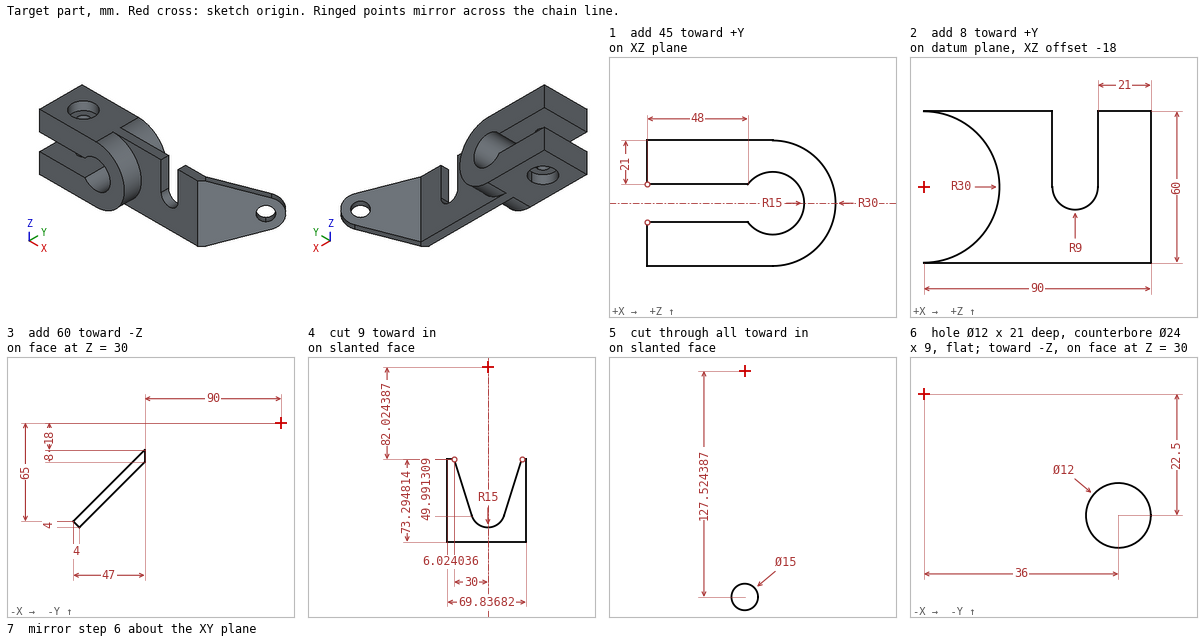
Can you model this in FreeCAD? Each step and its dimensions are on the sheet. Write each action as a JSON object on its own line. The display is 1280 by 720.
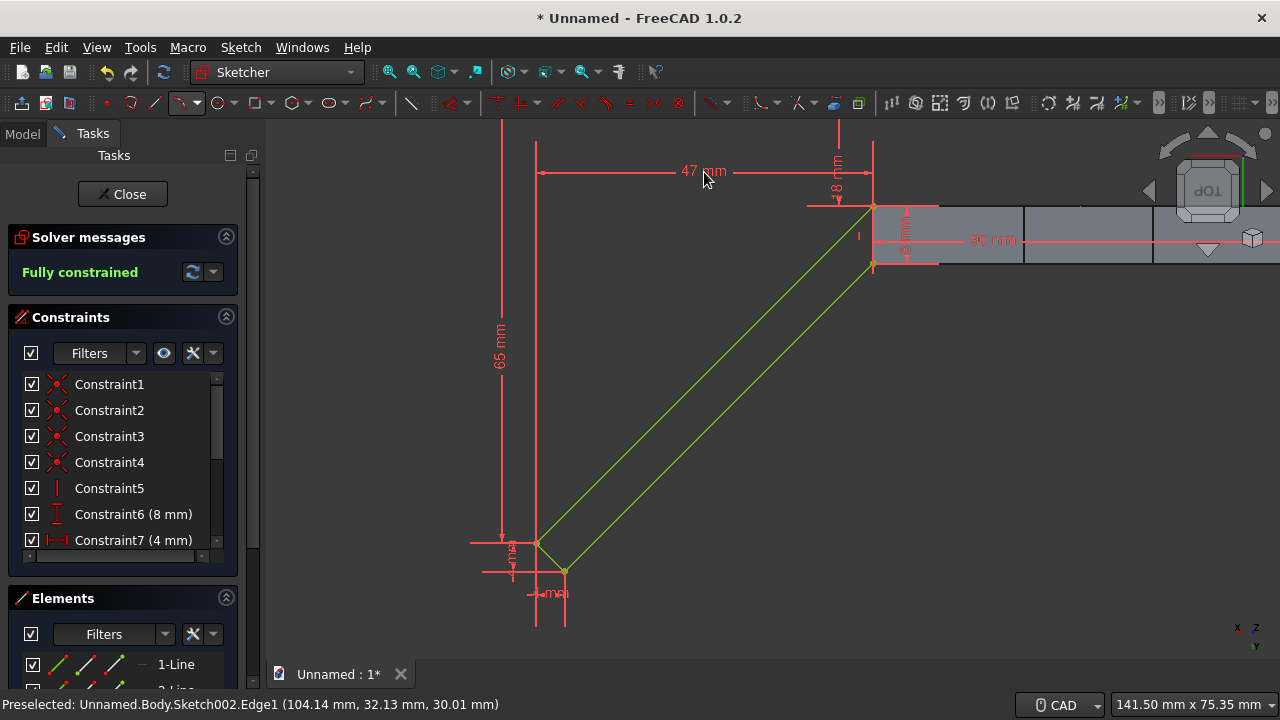
{"action": "left_click", "coordinate": [123, 194]}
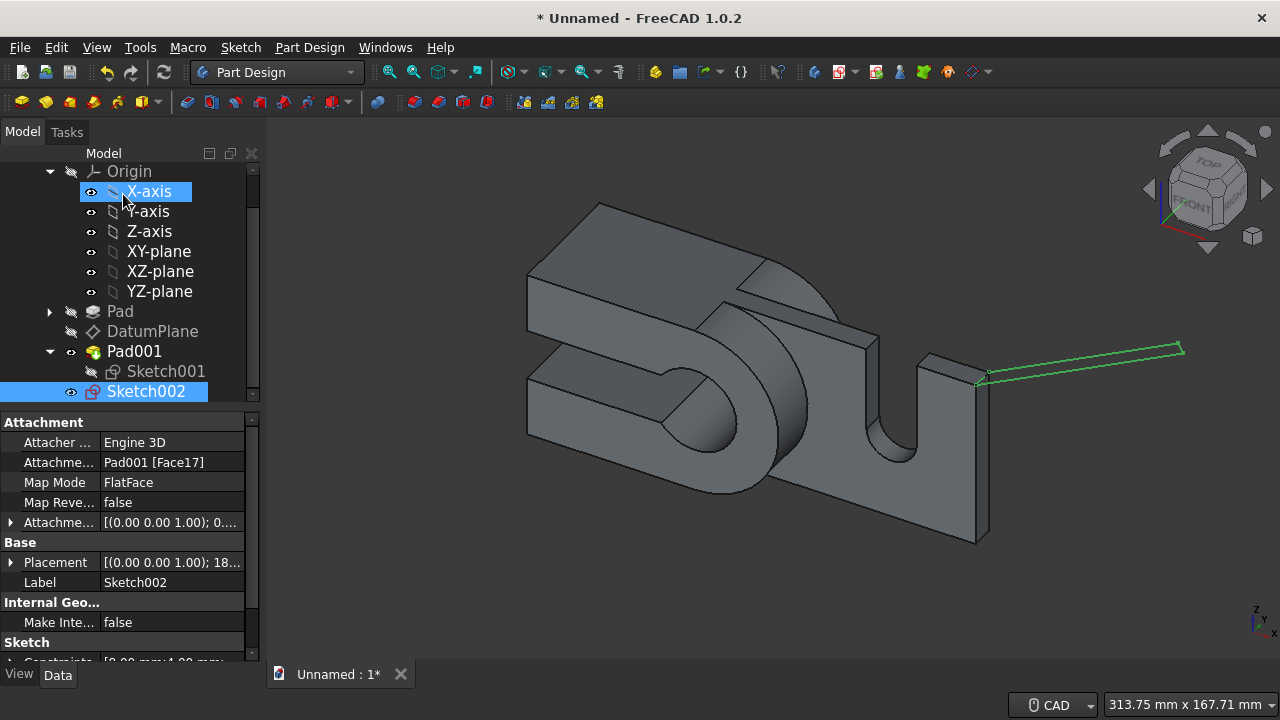
{"action": "left_click", "coordinate": [22, 102]}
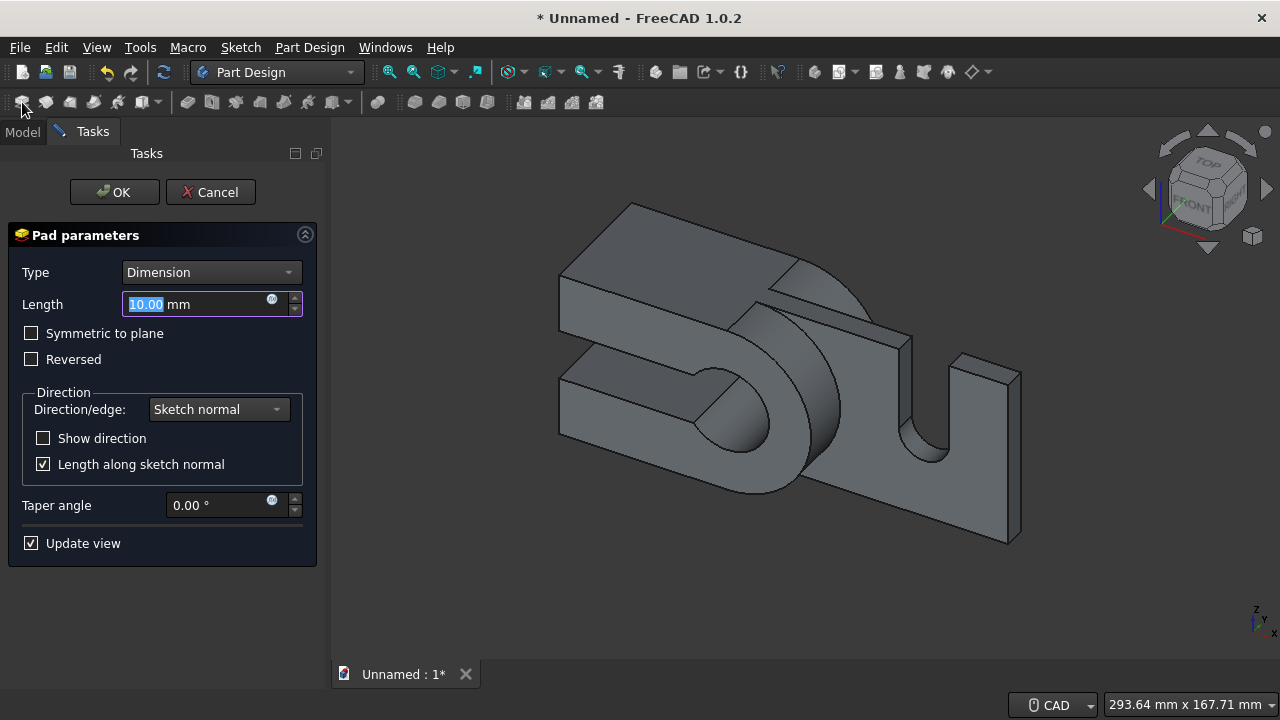
{"action": "type", "text": "60"}
{"action": "key", "text": "Tab"}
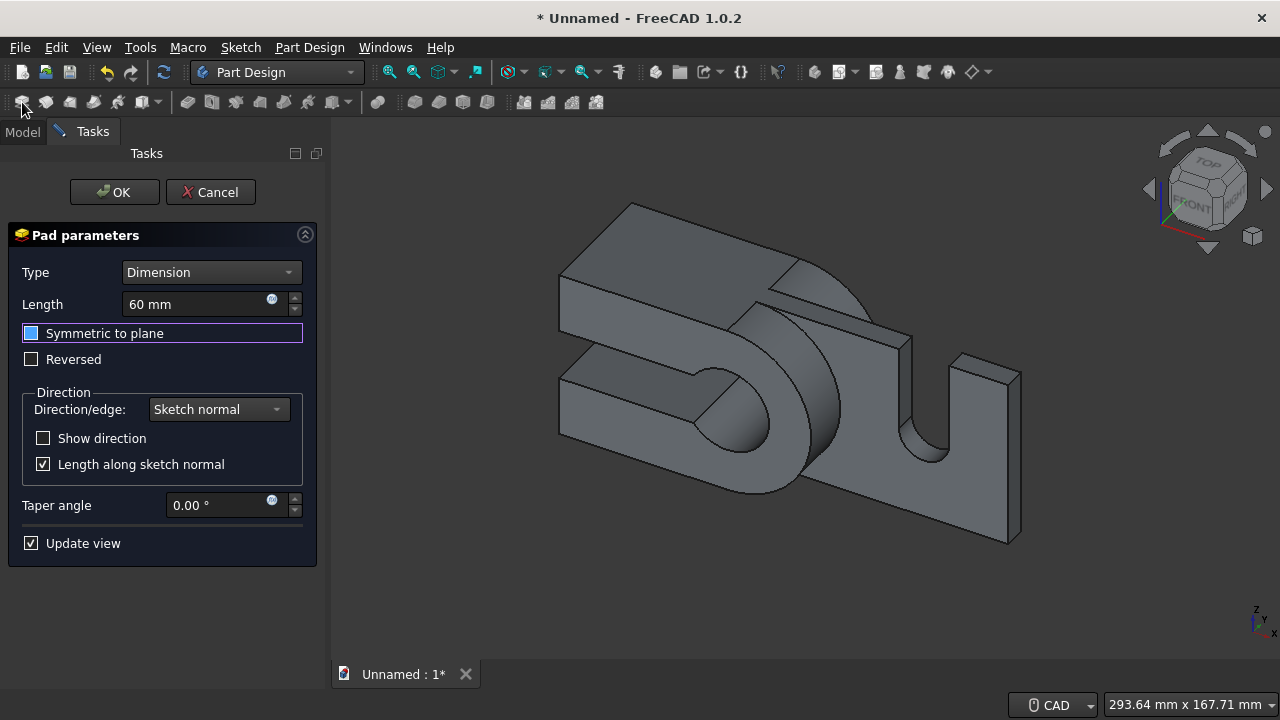
{"action": "left_click", "coordinate": [30, 359]}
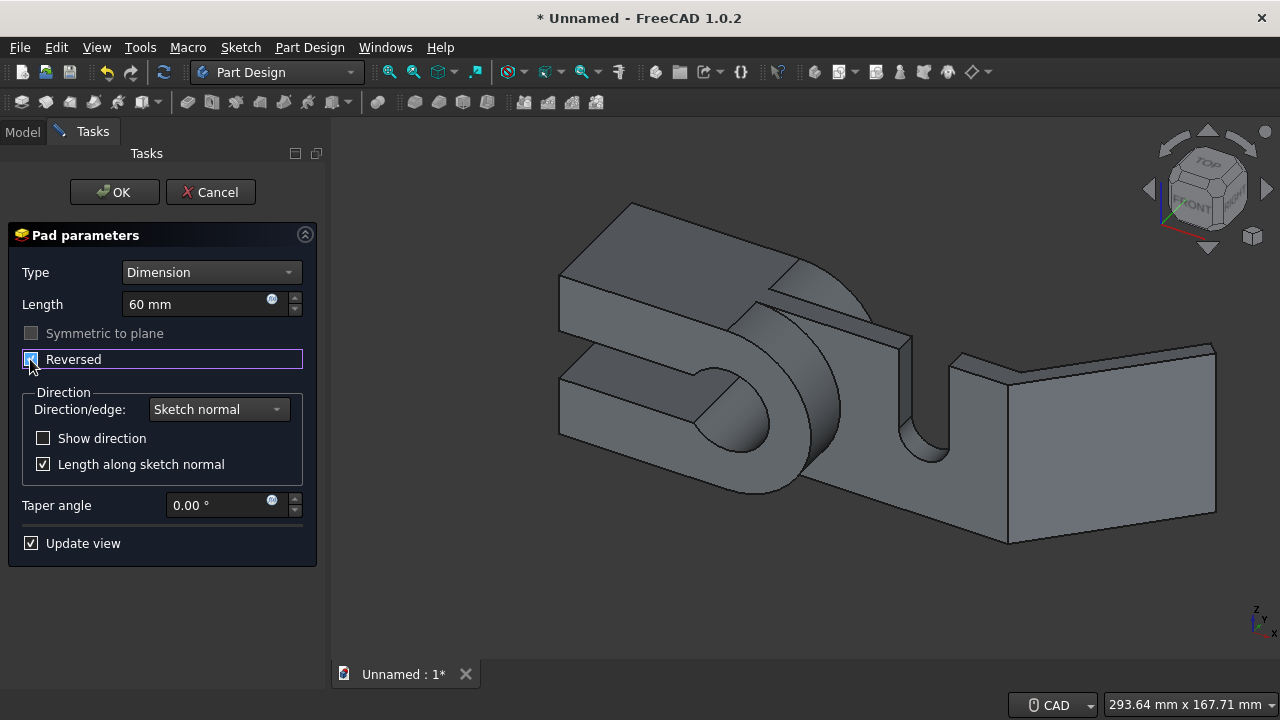
{"action": "left_click", "coordinate": [115, 192]}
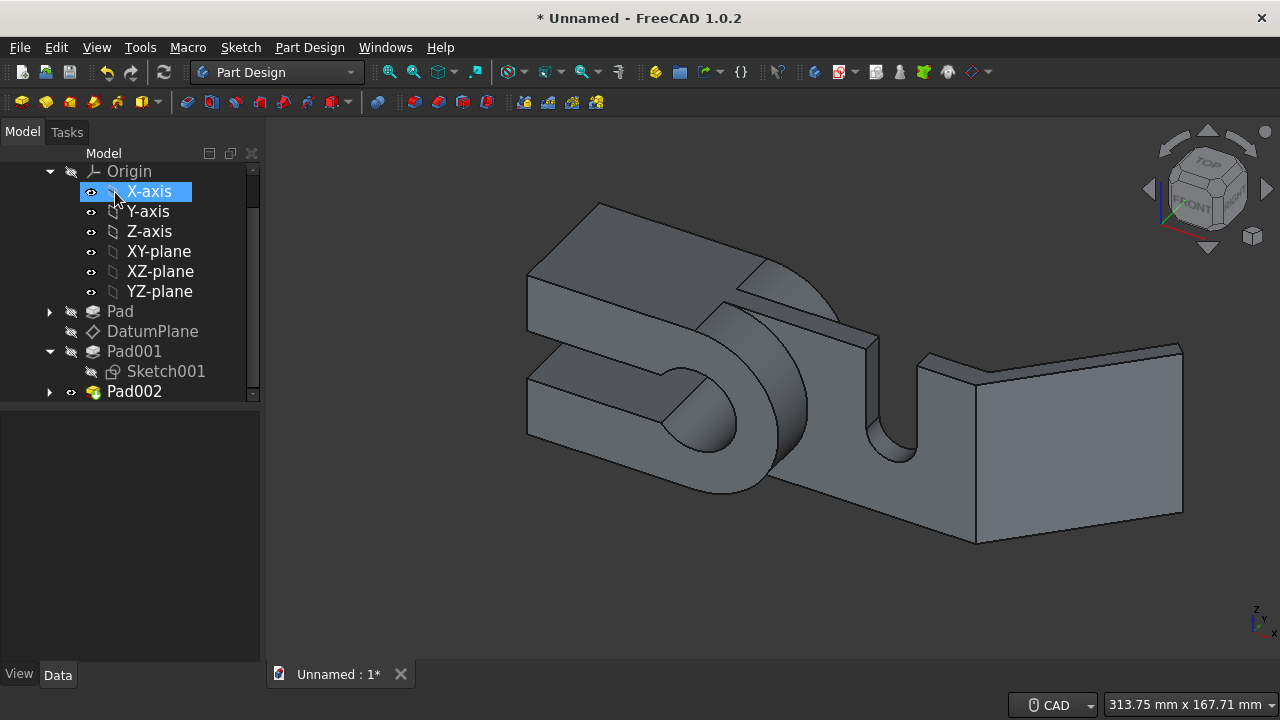
{"action": "key", "text": "4"}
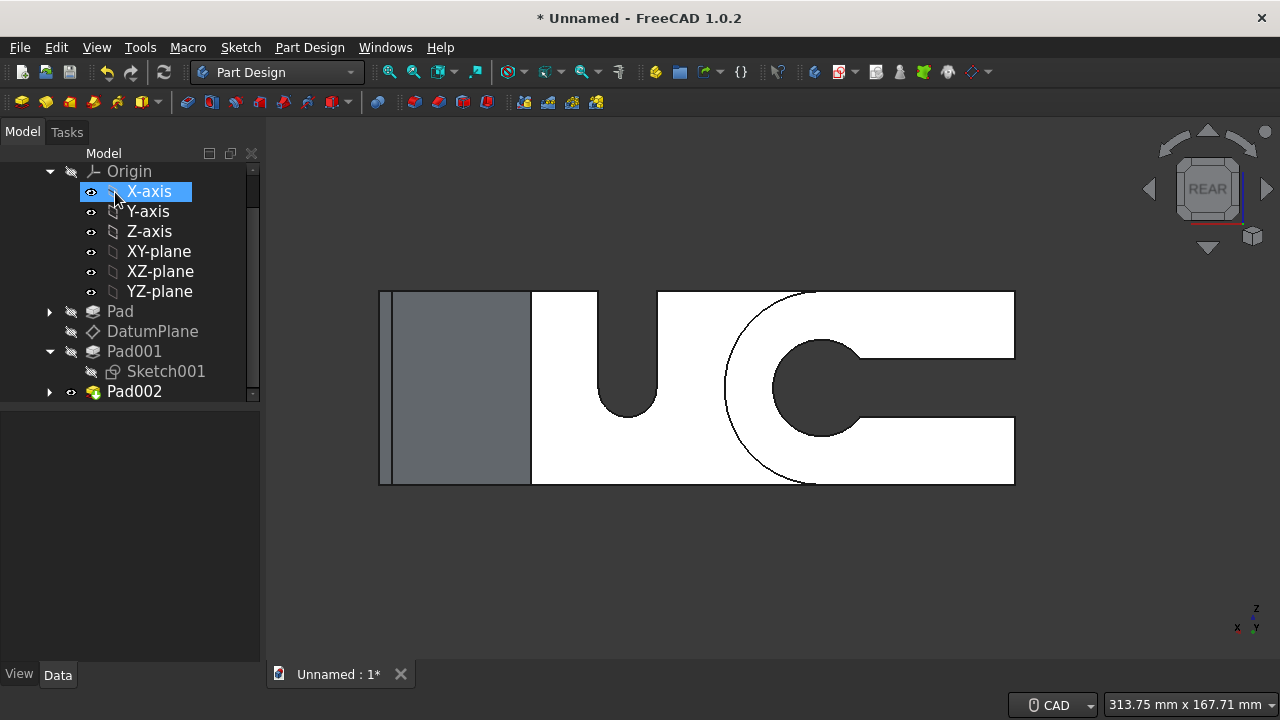
{"action": "left_click", "coordinate": [461, 387]}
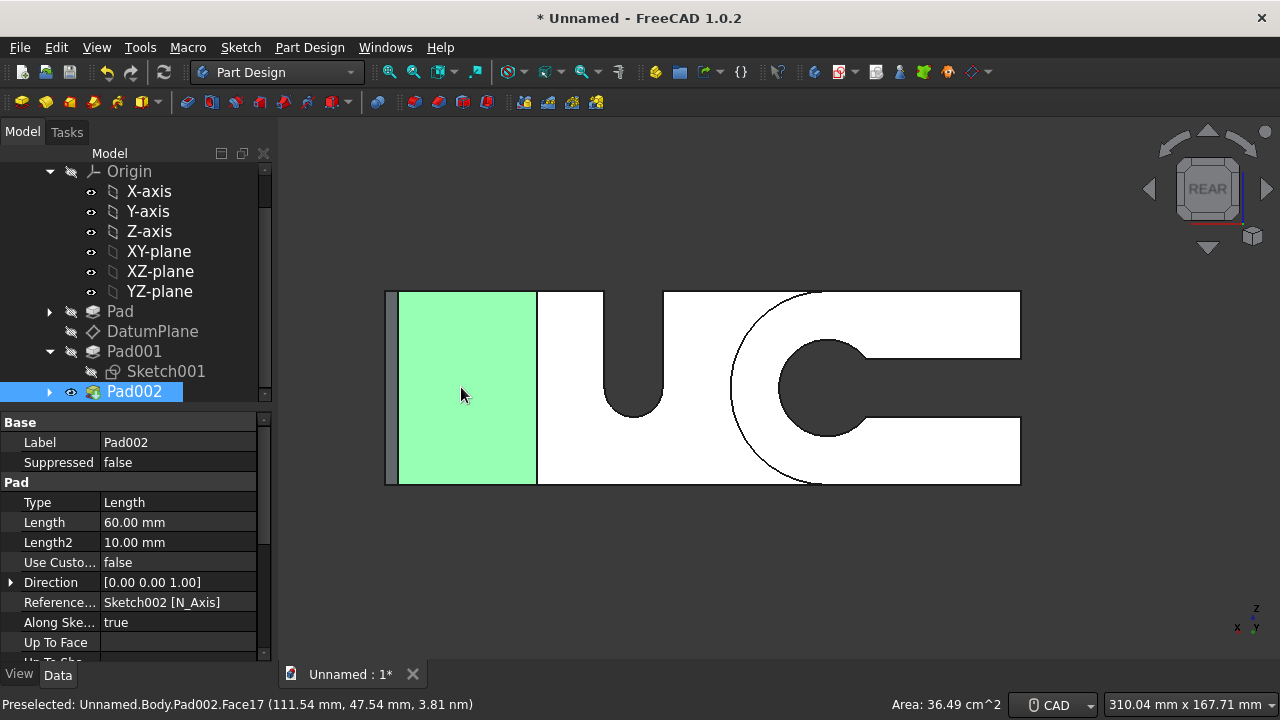
{"action": "left_click", "coordinate": [840, 72]}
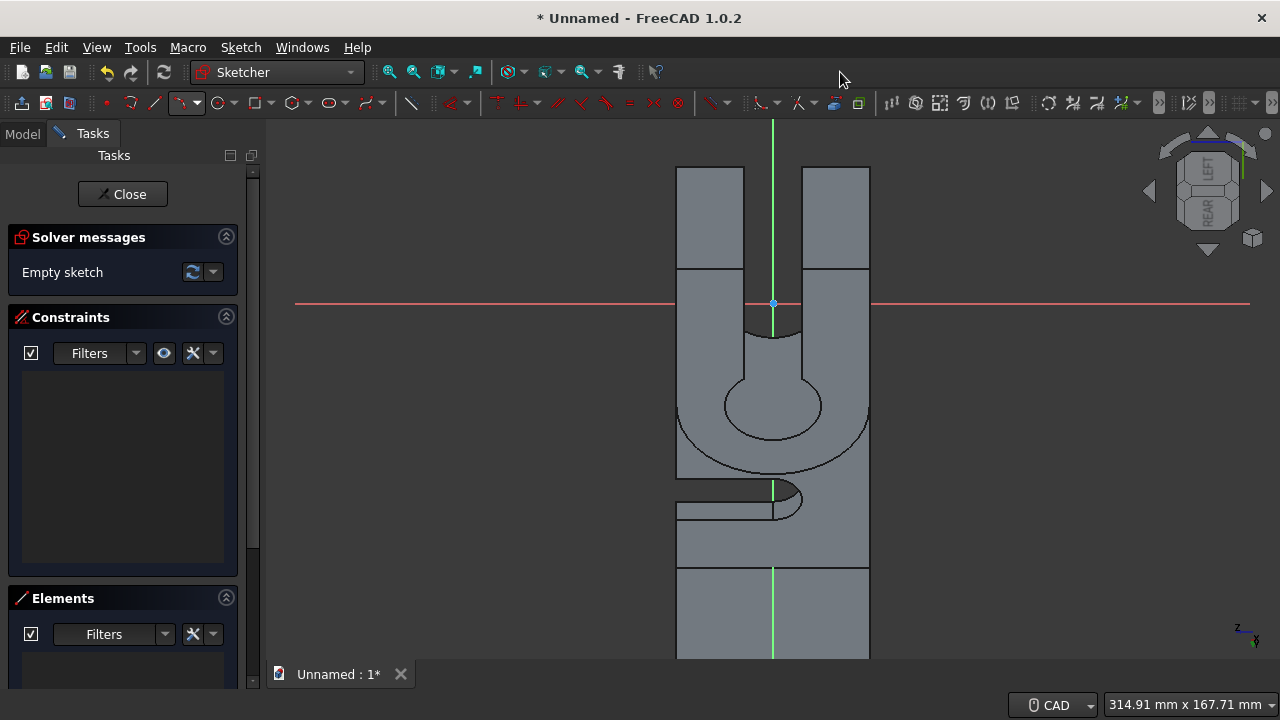
{"action": "left_click", "coordinate": [70, 104]}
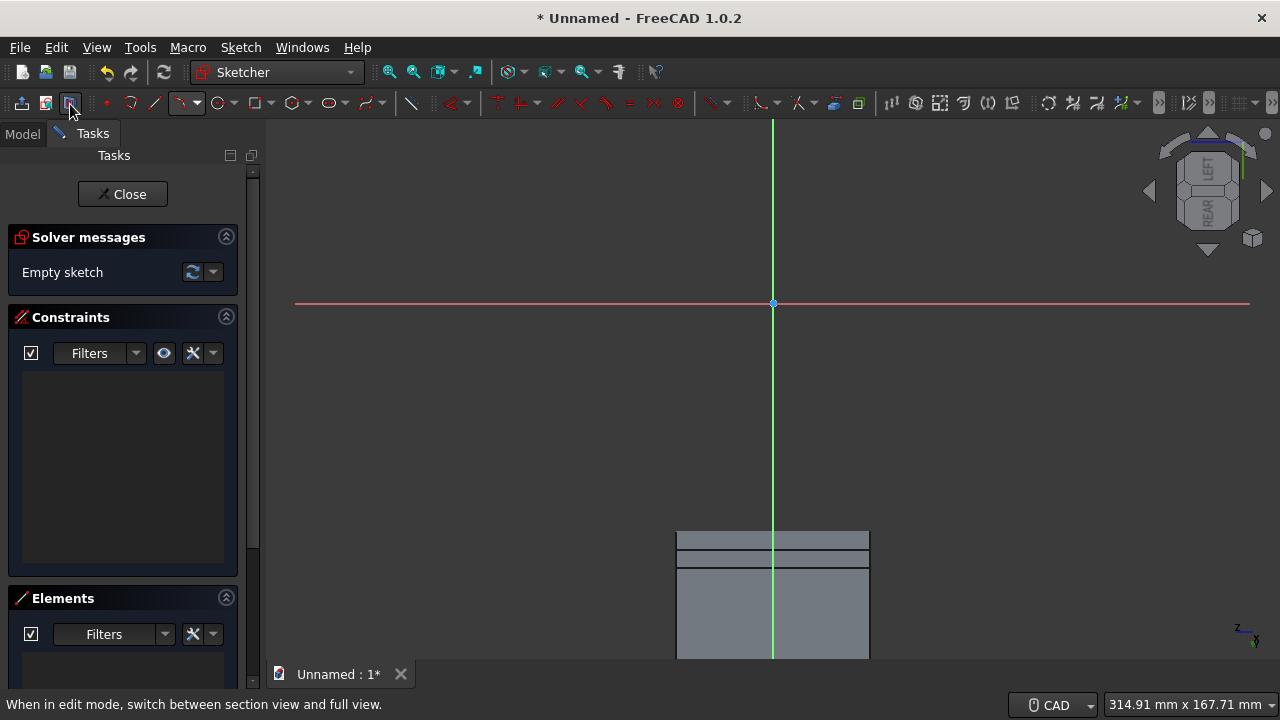
{"action": "scroll", "coordinate": [572, 147], "scroll_direction": "down", "scroll_amount": 2}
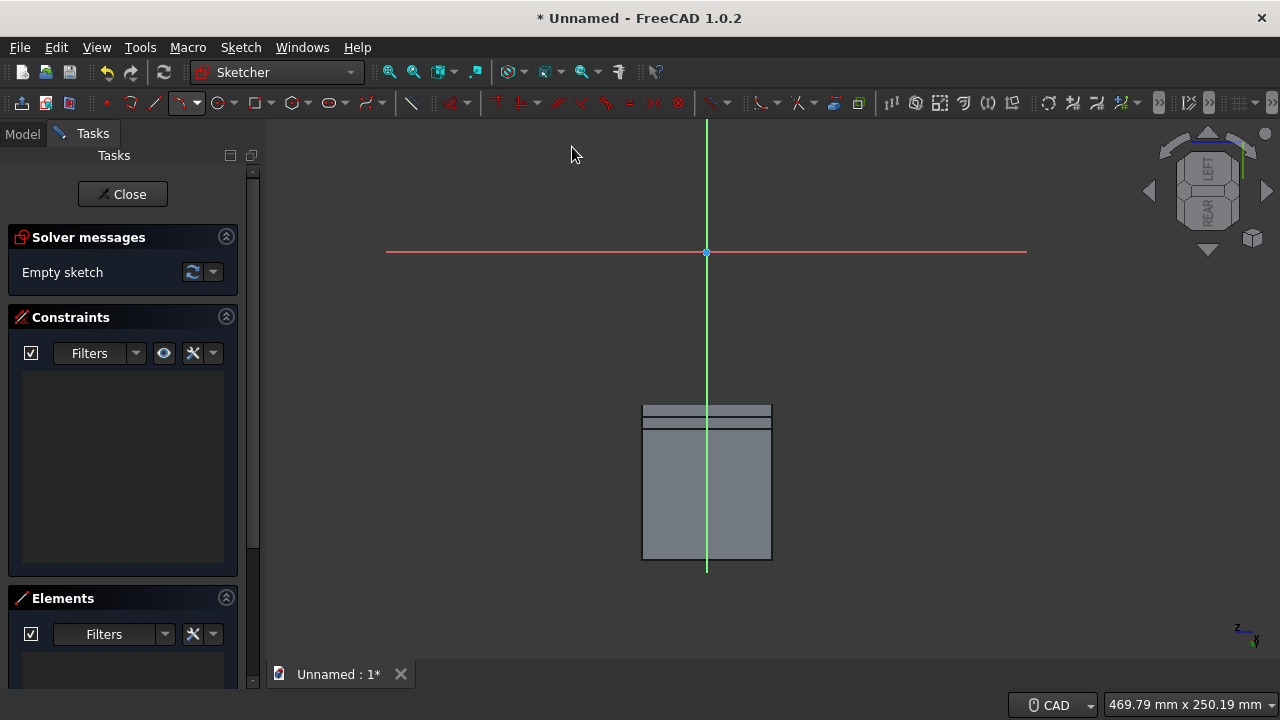
{"action": "left_click", "coordinate": [132, 104]}